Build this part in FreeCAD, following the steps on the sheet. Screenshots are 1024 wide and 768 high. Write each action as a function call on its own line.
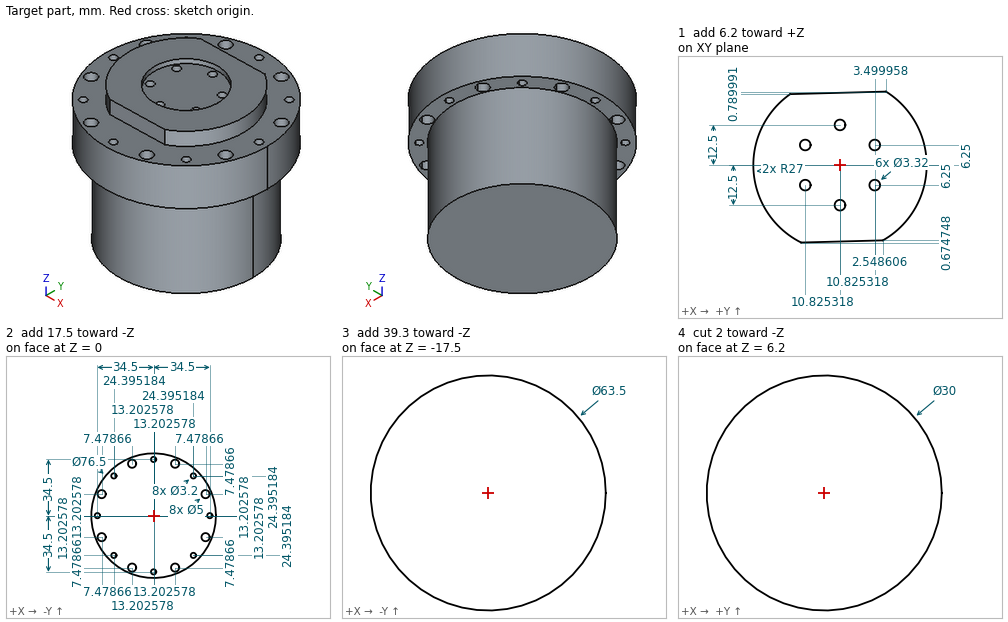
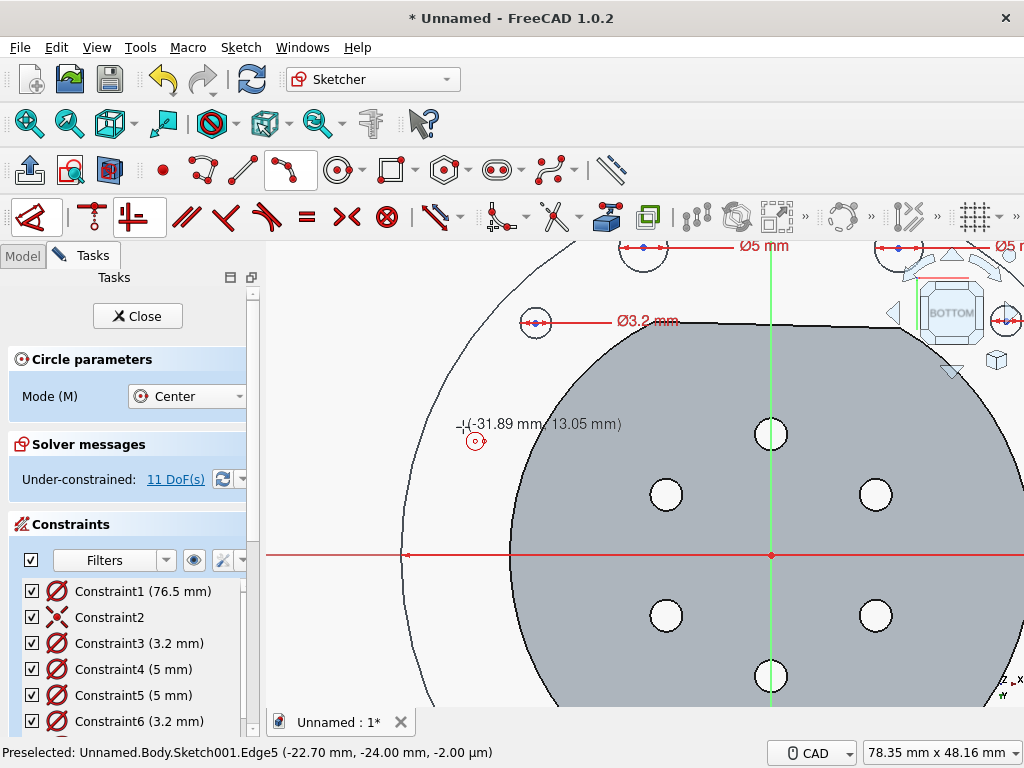
click(463, 428)
move(480, 410)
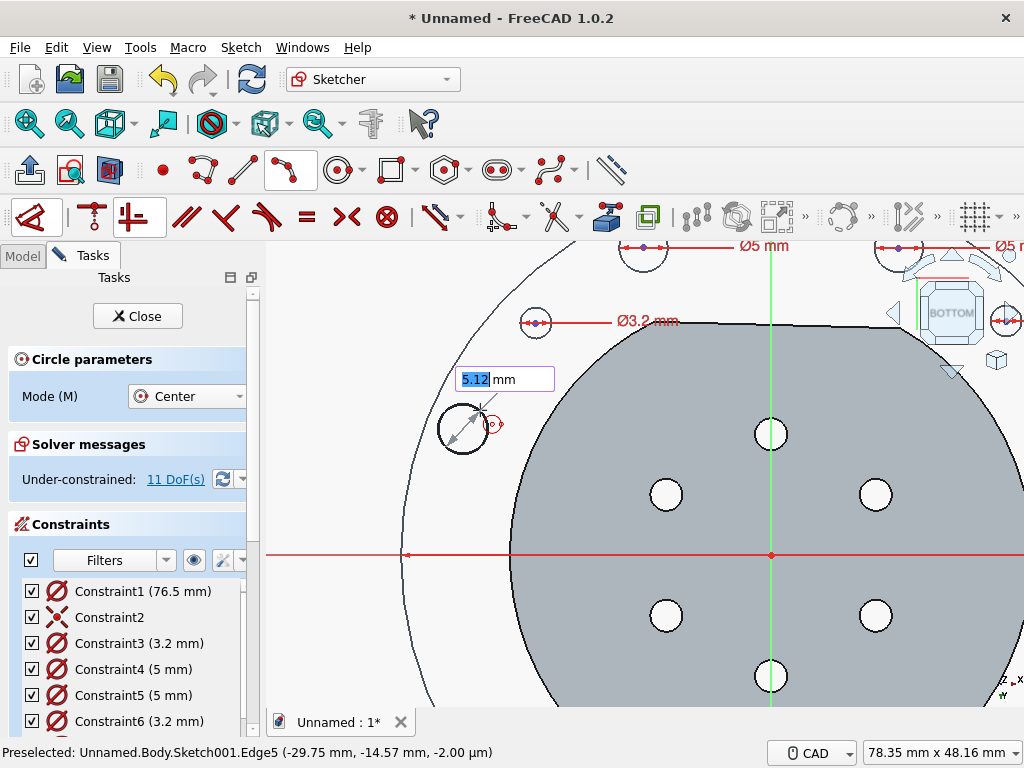
text(5)
key(Return)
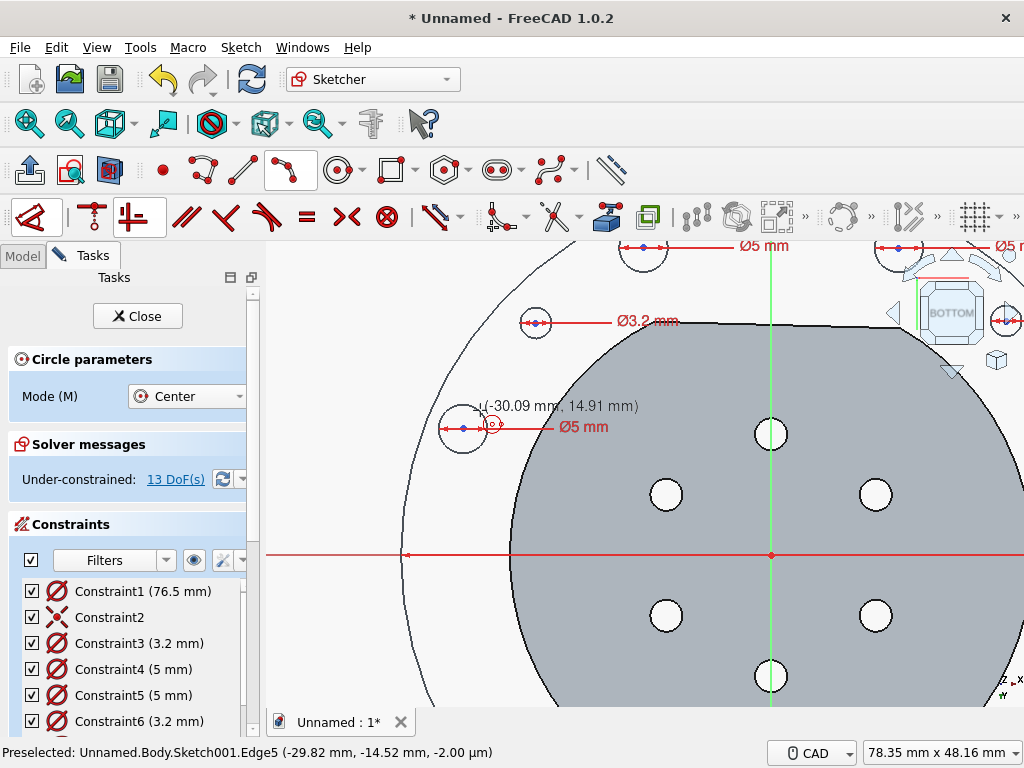
scroll(463, 427, down, 5)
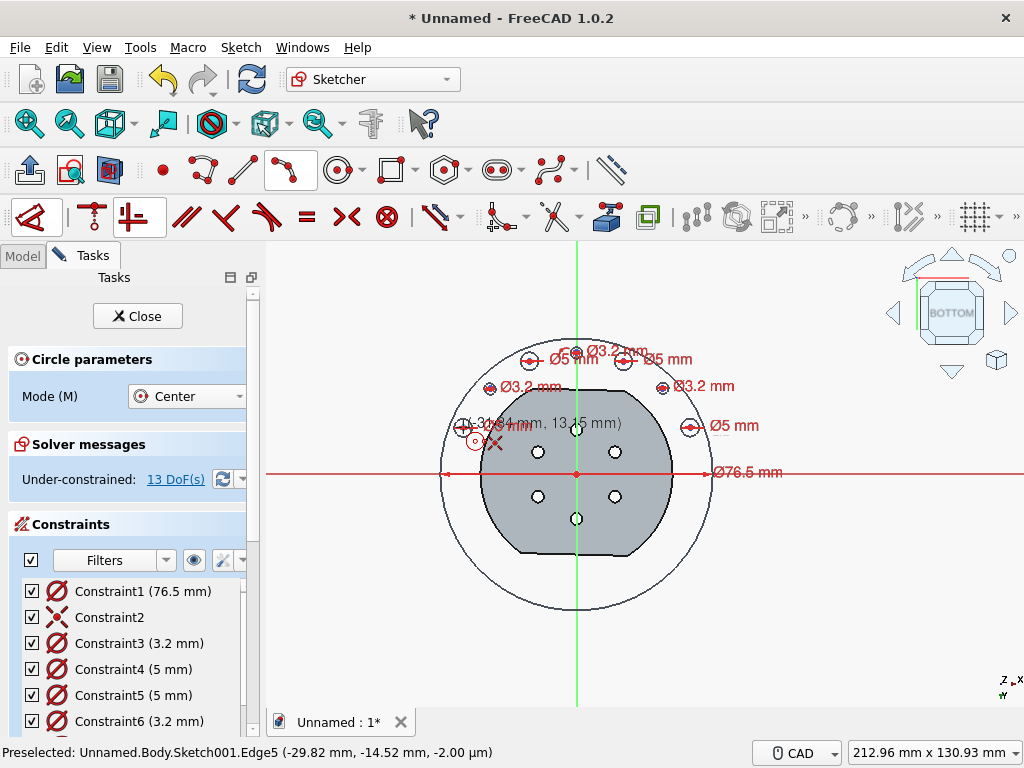
scroll(699, 474, up, 7)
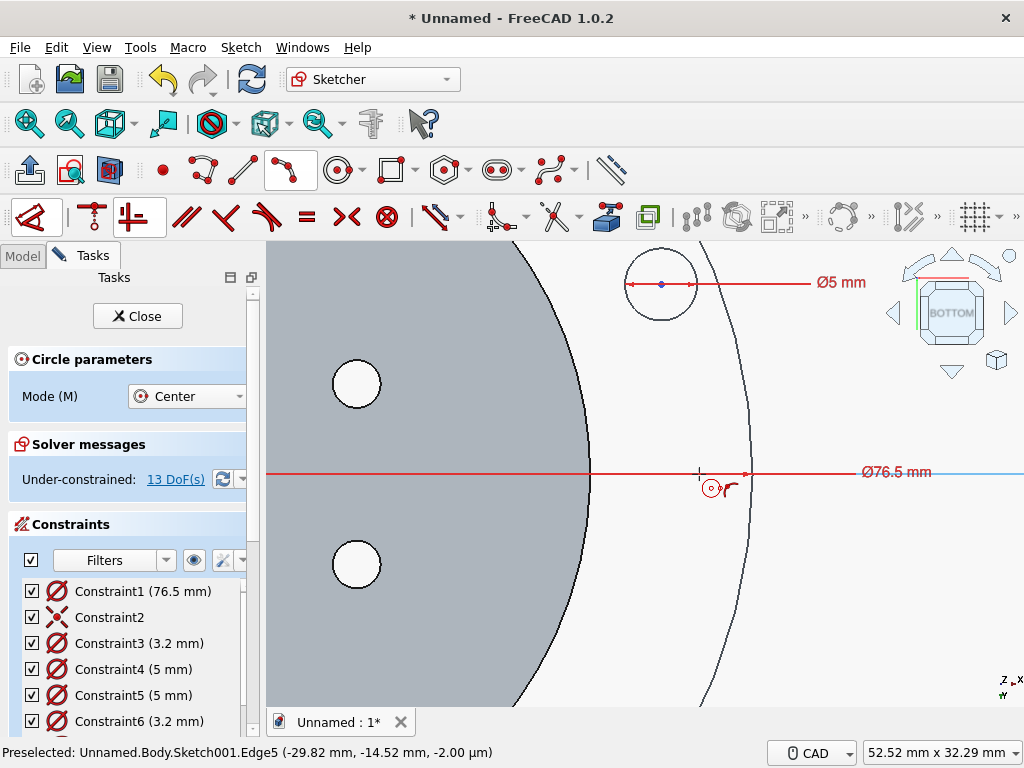
scroll(700, 474, down, 7)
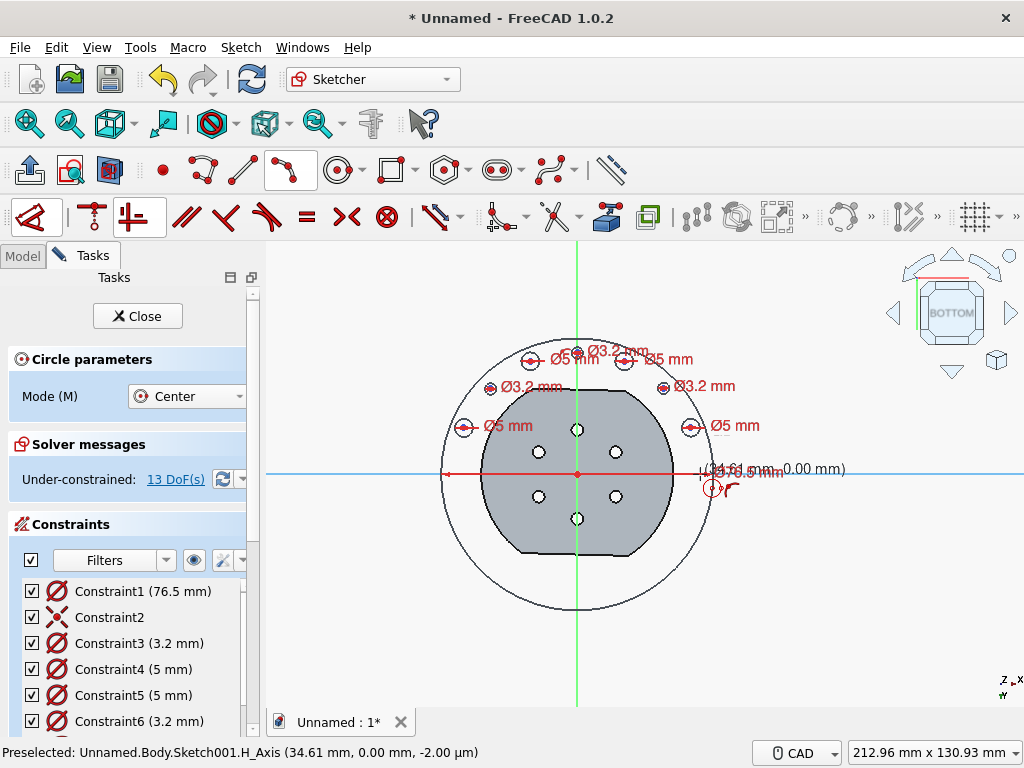
click(700, 474)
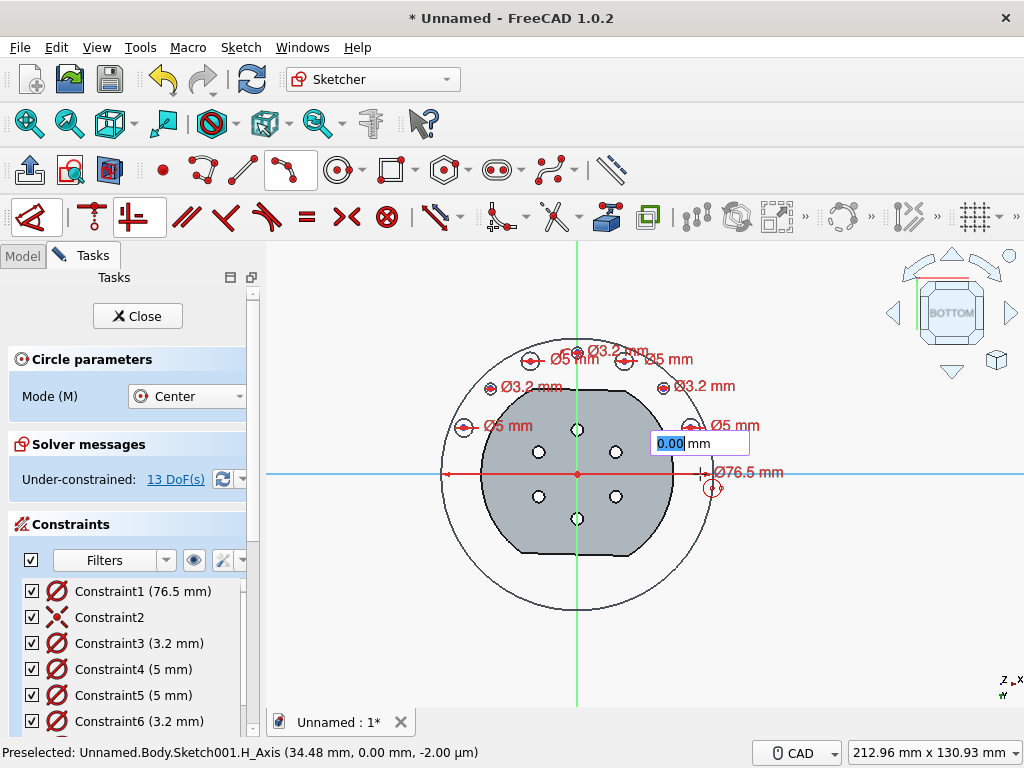
scroll(698, 480, up, 6)
move(697, 478)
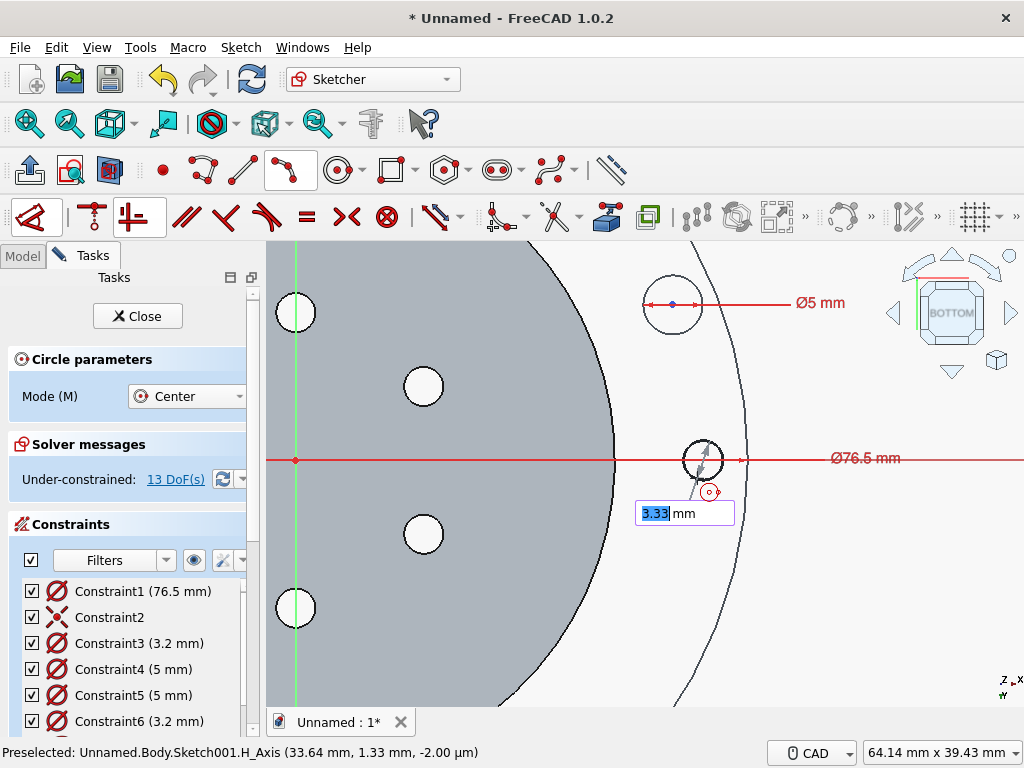
text(3.2)
key(Return)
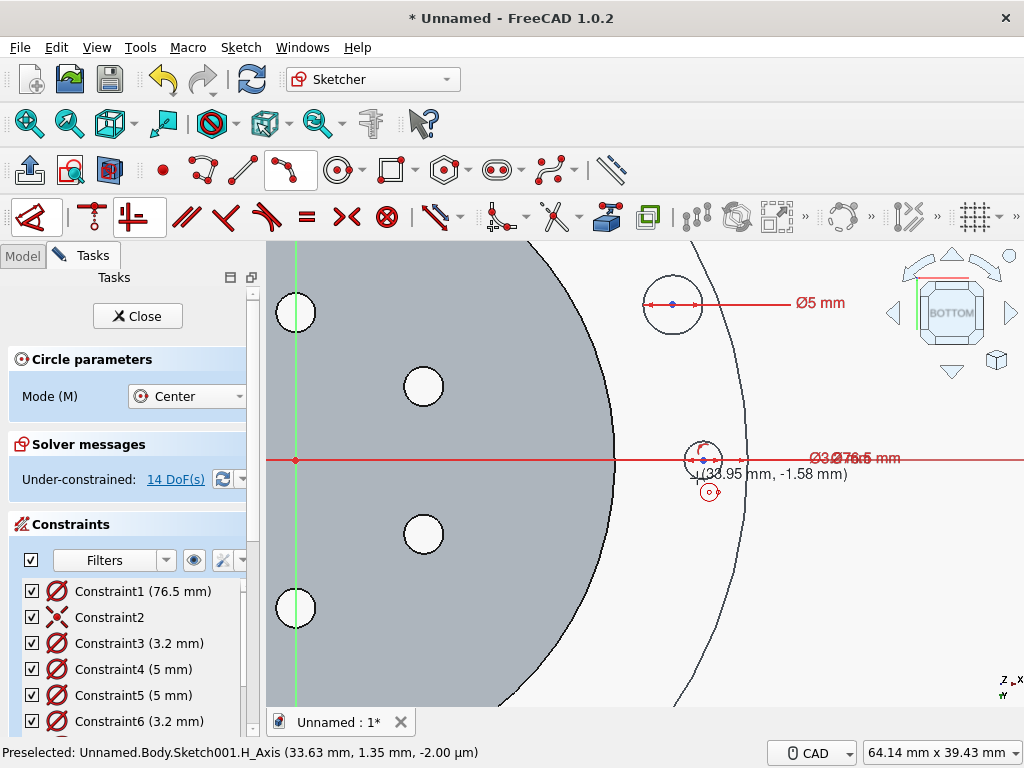
click(672, 616)
move(693, 595)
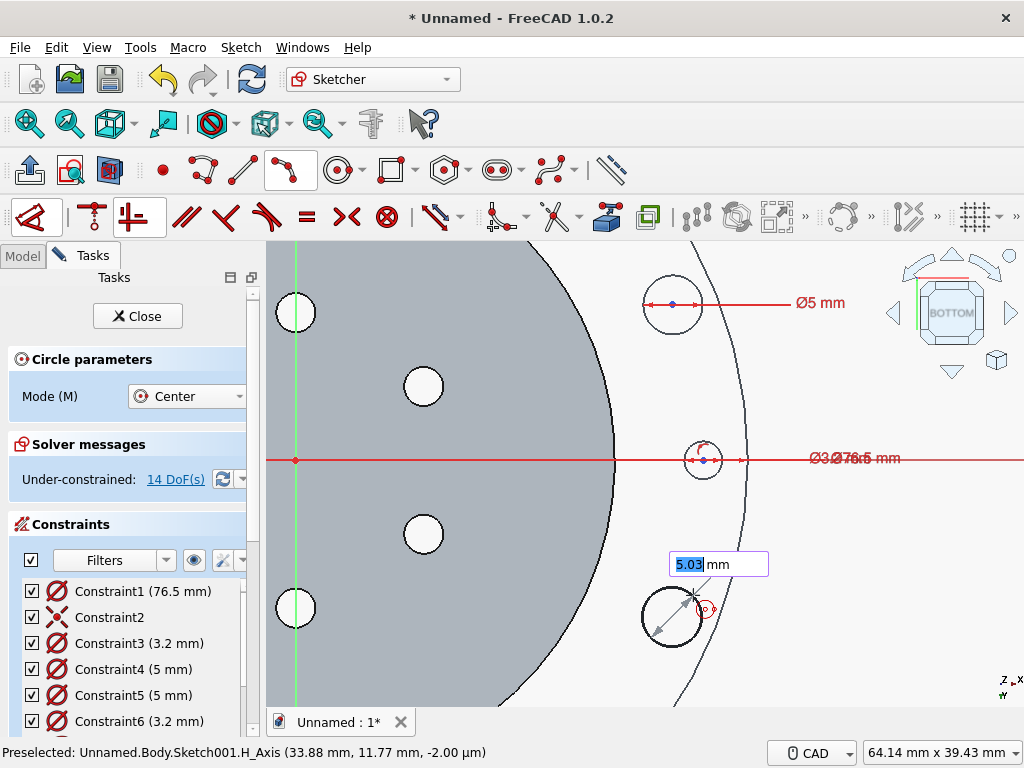
text(5)
key(Return)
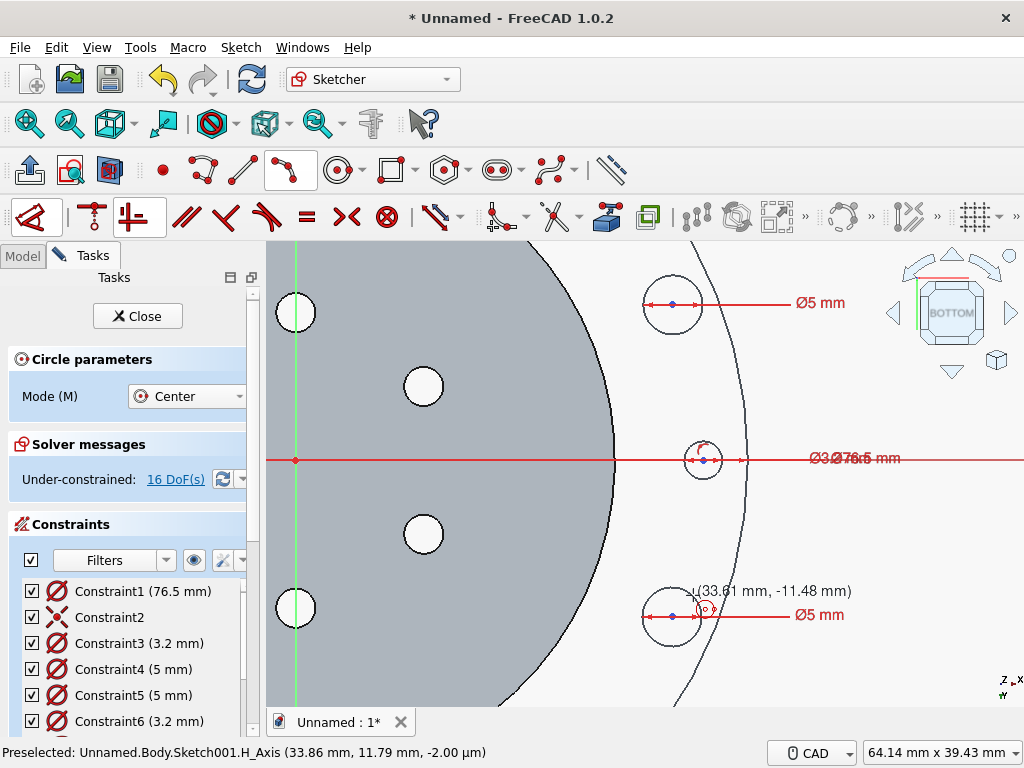
scroll(697, 480, down, 6)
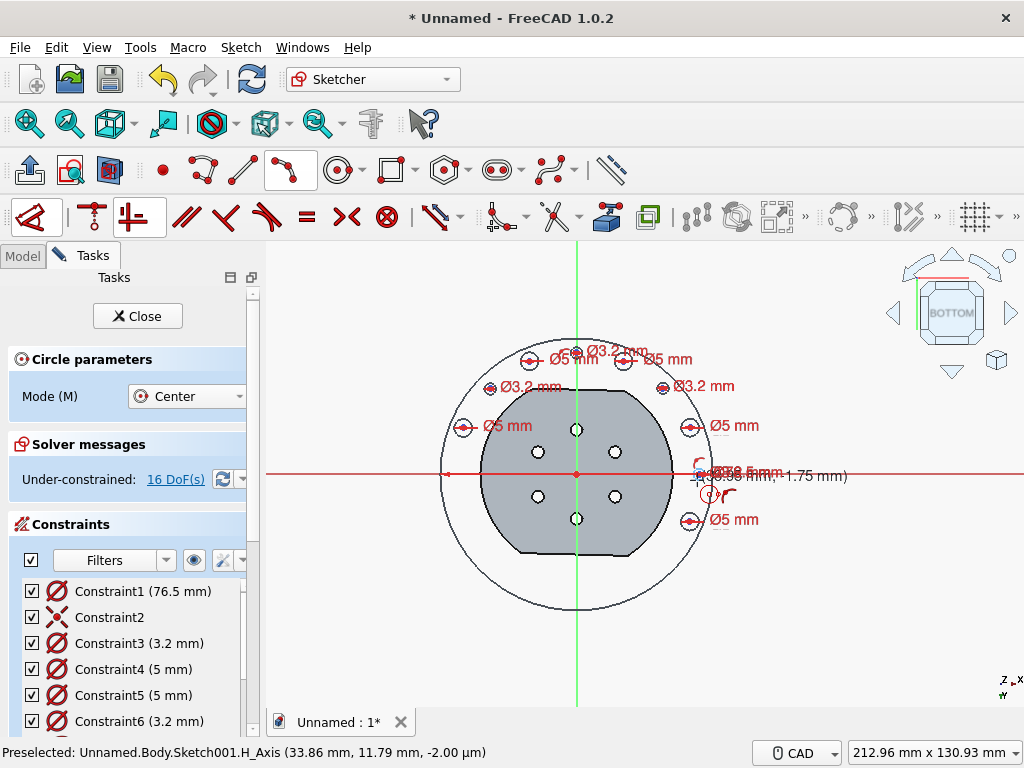
scroll(663, 561, up, 7)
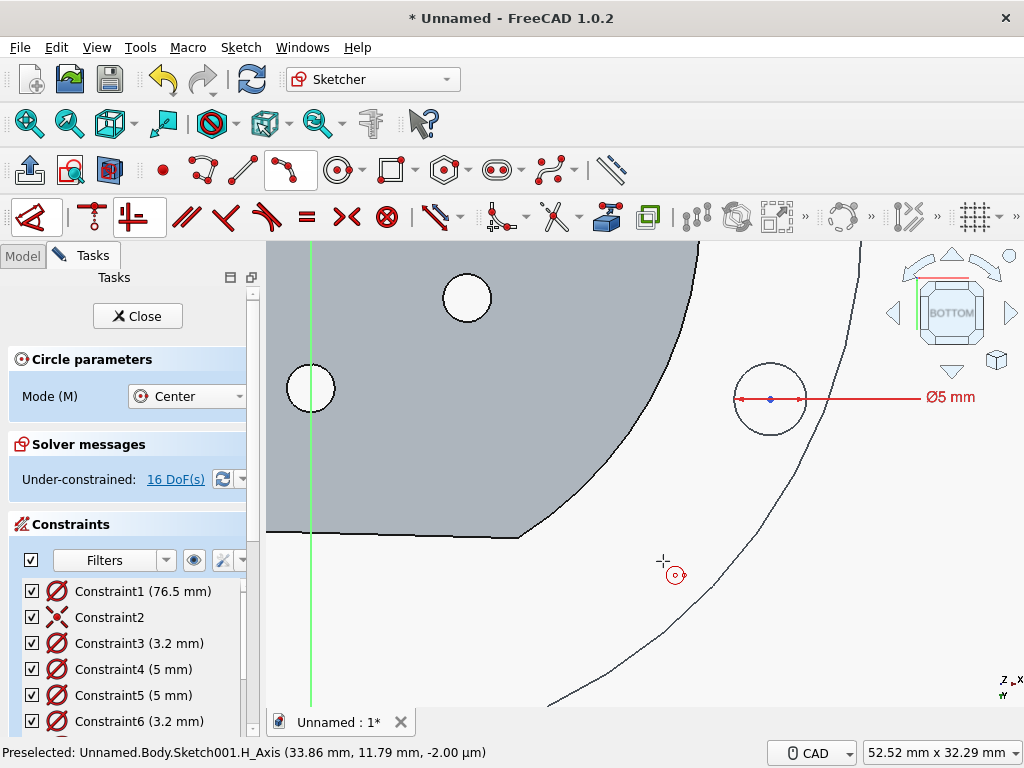
scroll(663, 561, down, 7)